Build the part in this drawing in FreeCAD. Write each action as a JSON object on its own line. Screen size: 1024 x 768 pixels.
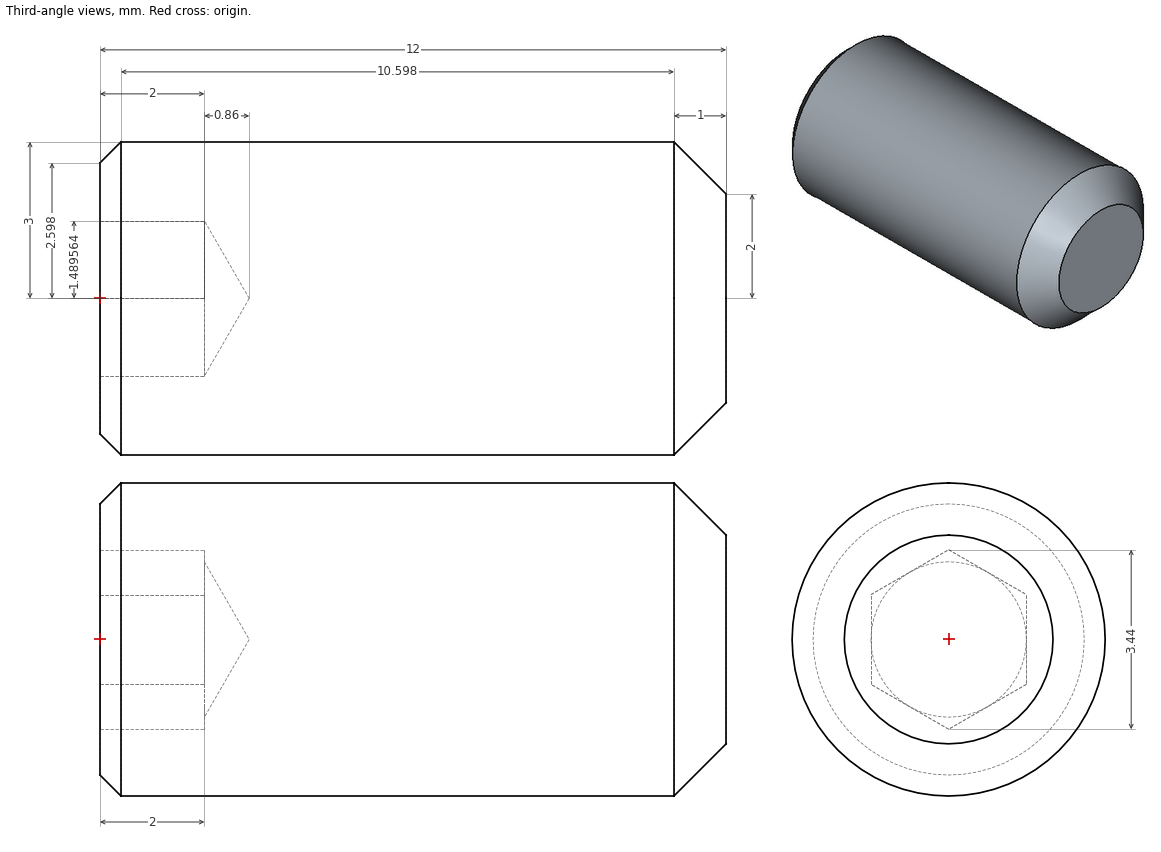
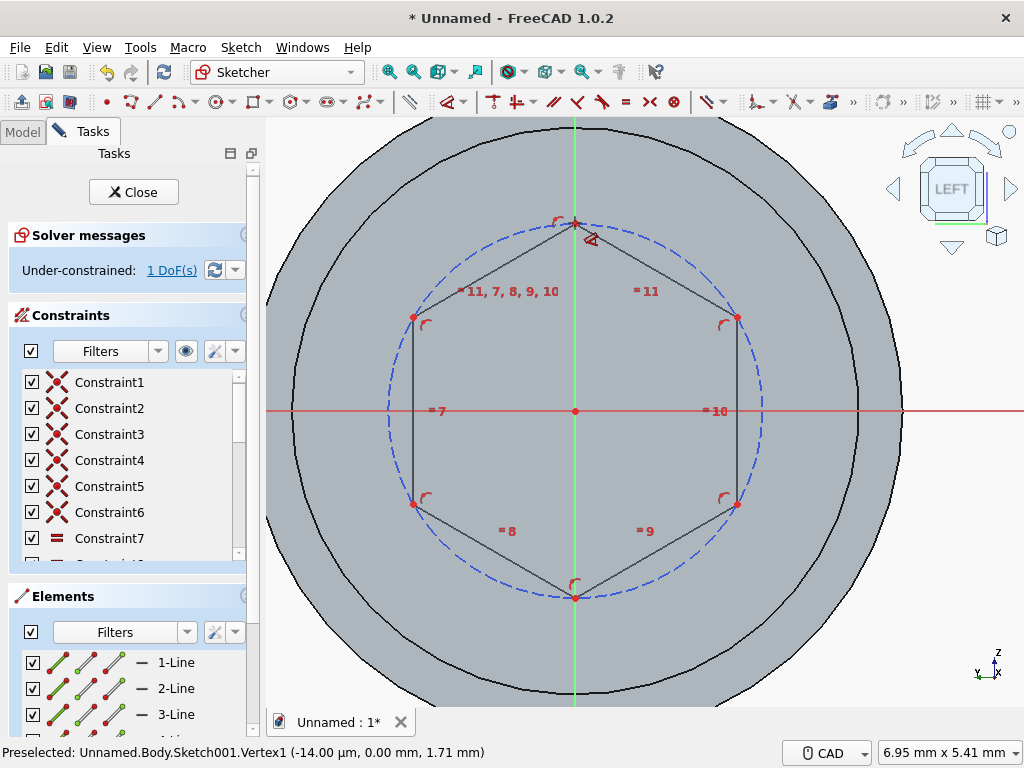
{"action": "left_click", "coordinate": [575, 598]}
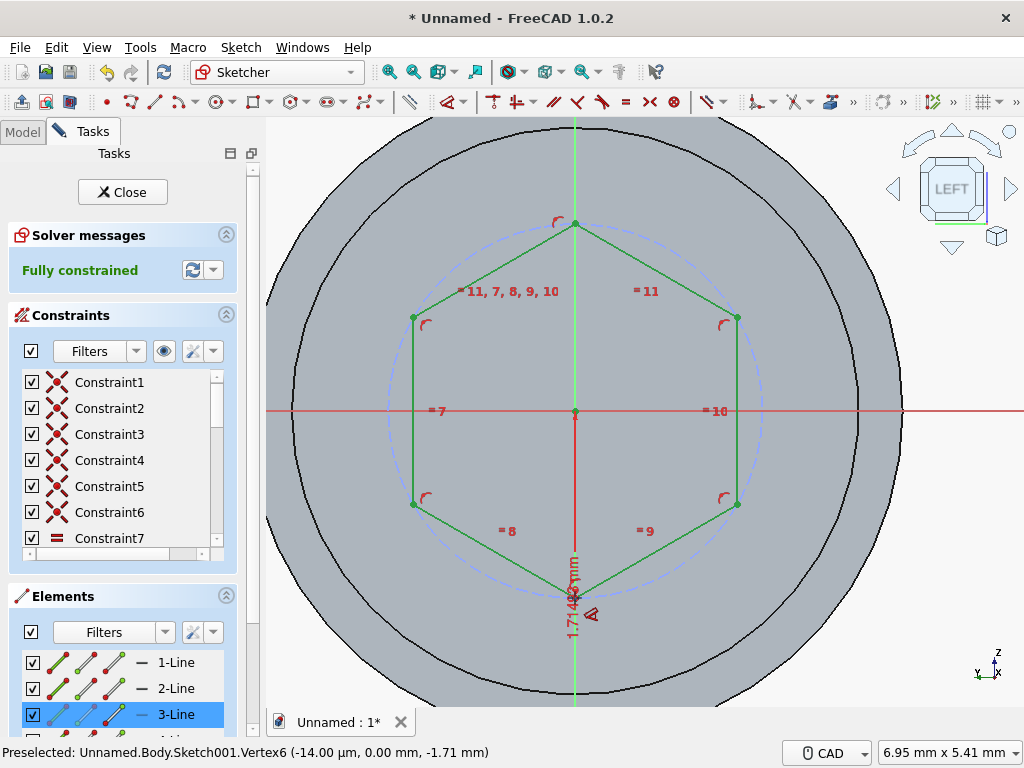
{"action": "left_click", "coordinate": [575, 224]}
{"action": "left_click", "coordinate": [609, 325]}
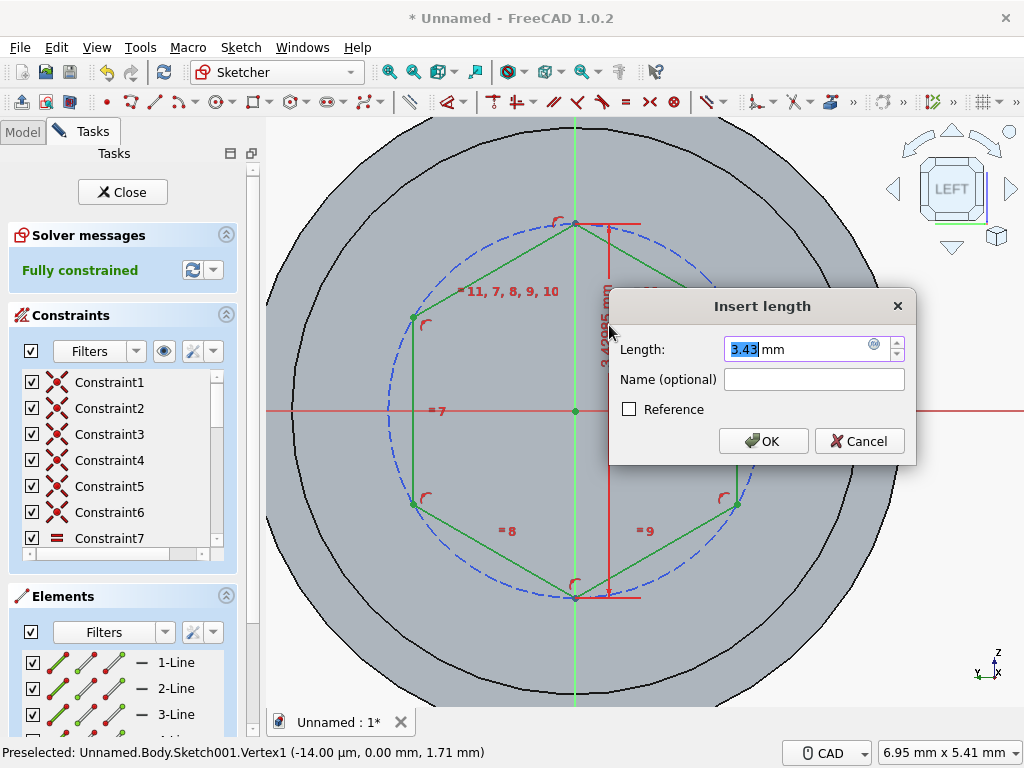
{"action": "type", "text": "3.44"}
{"action": "key", "text": "Return"}
{"action": "key", "text": "Escape"}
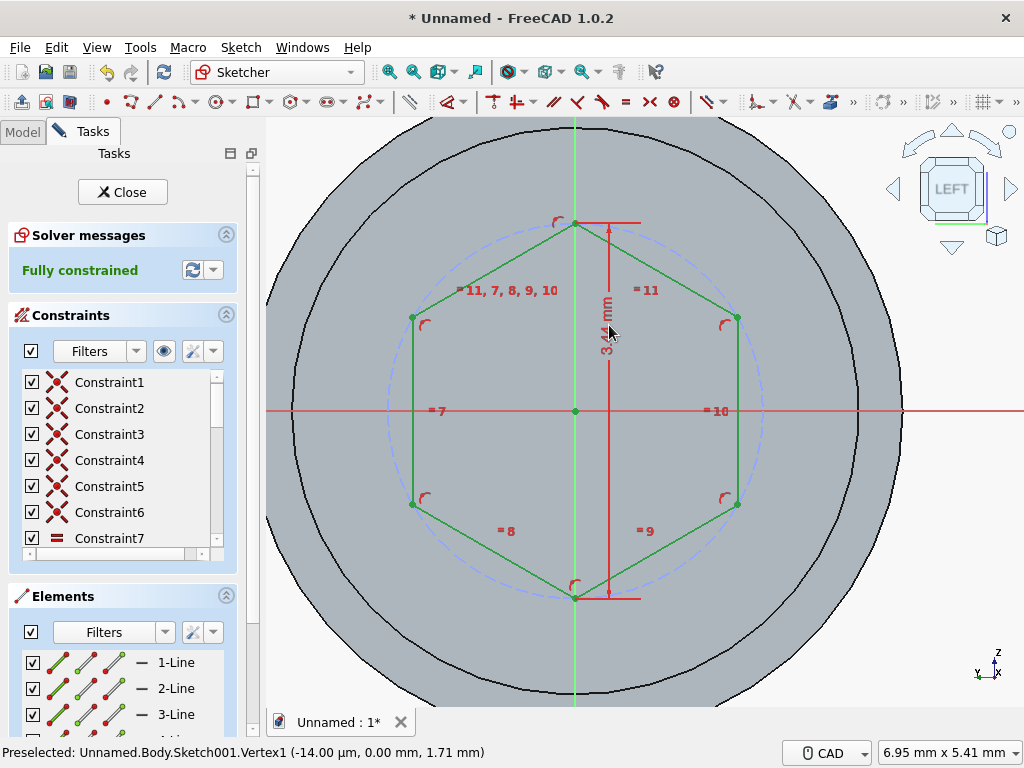
{"action": "left_click", "coordinate": [123, 192]}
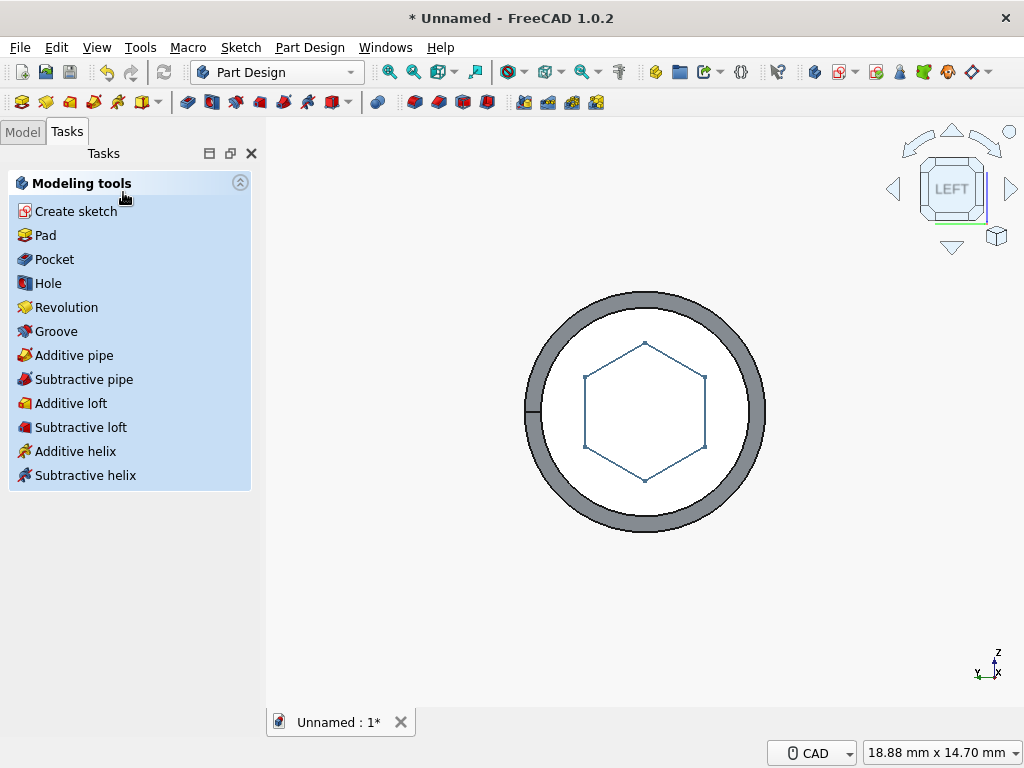
{"action": "left_click", "coordinate": [188, 102]}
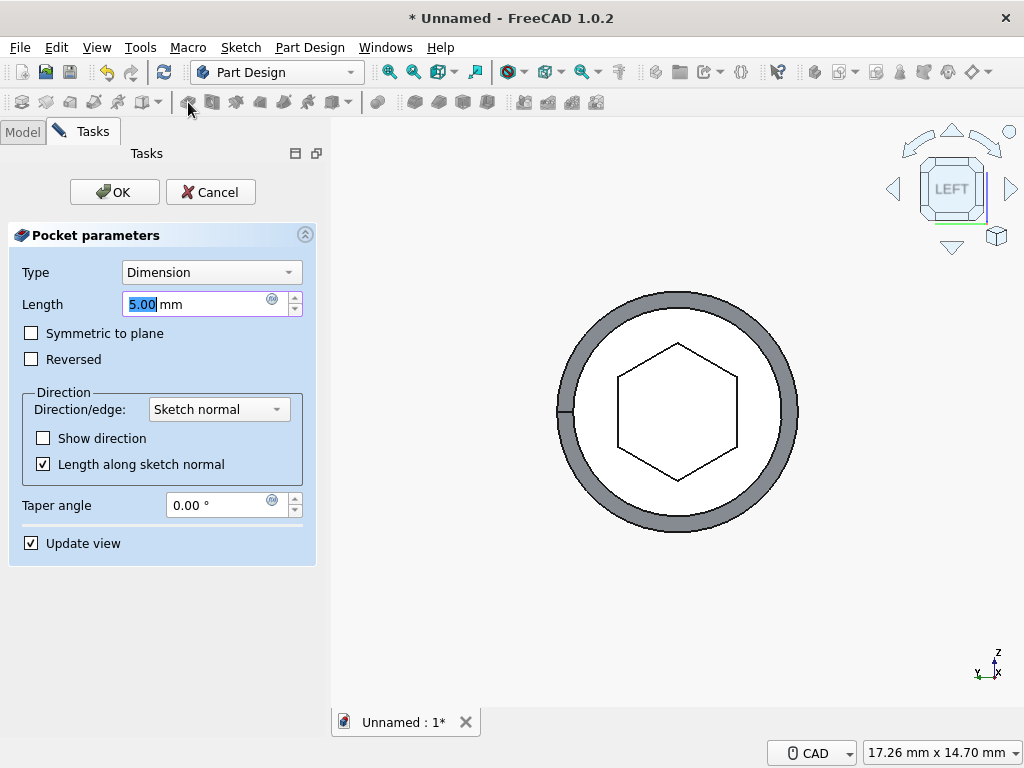
{"action": "type", "text": "2"}
{"action": "key", "text": "Tab"}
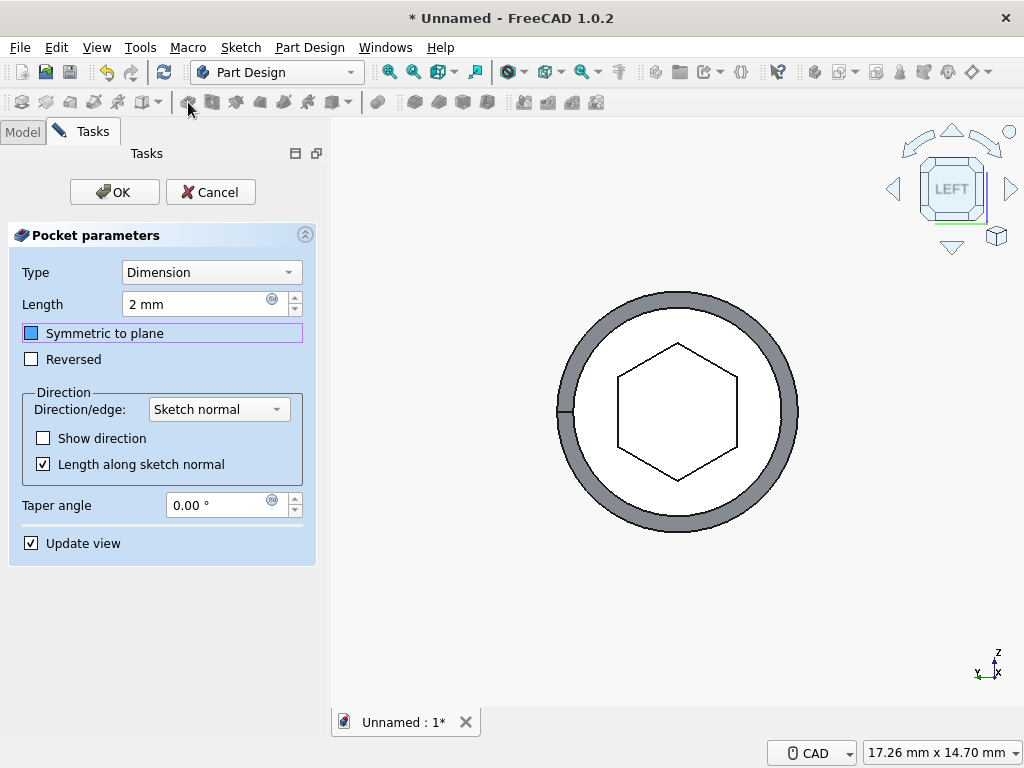
{"action": "left_click", "coordinate": [115, 192]}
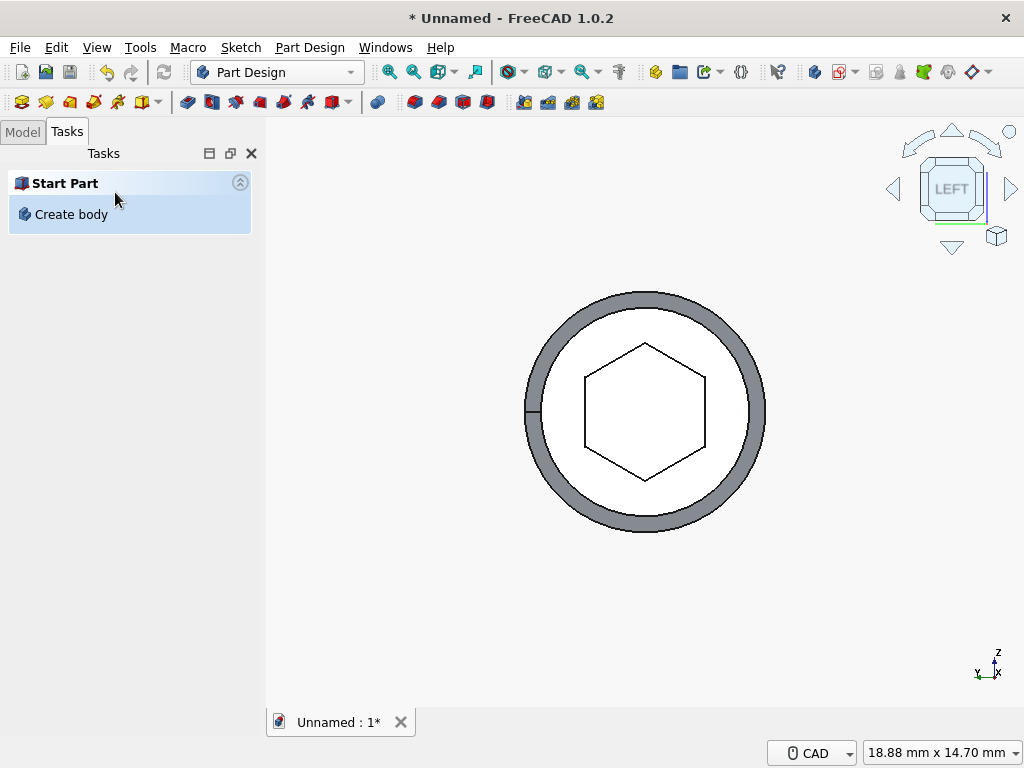
{"action": "left_click", "coordinate": [390, 72]}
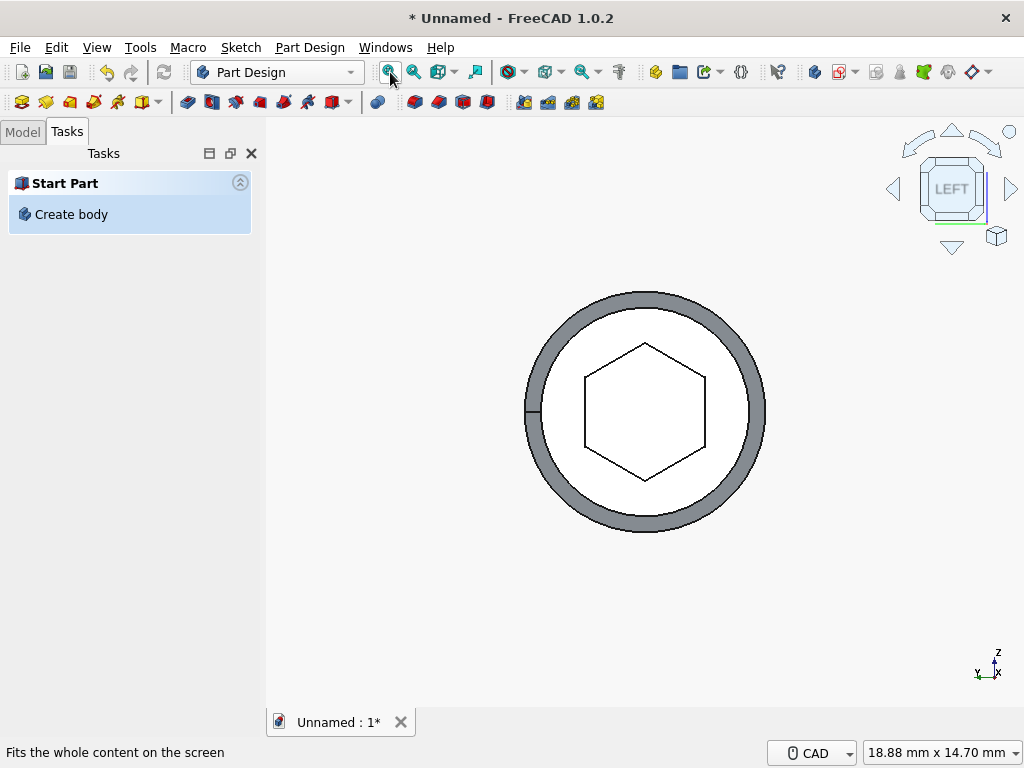
{"action": "left_click", "coordinate": [840, 72]}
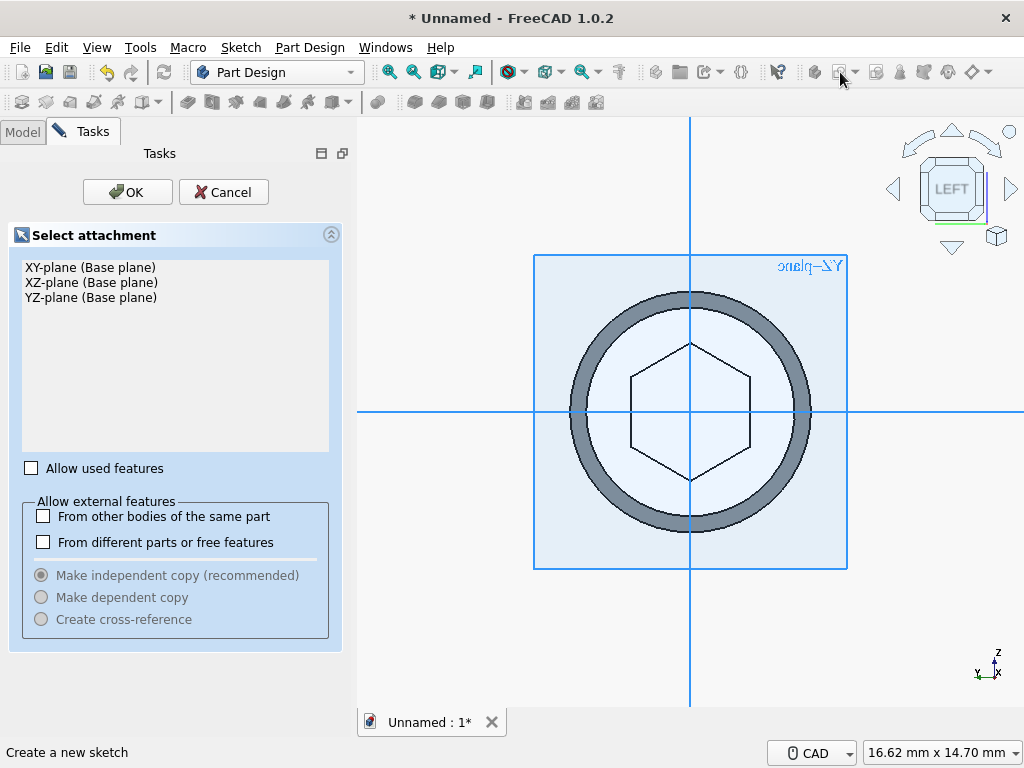
{"action": "left_click", "coordinate": [82, 268]}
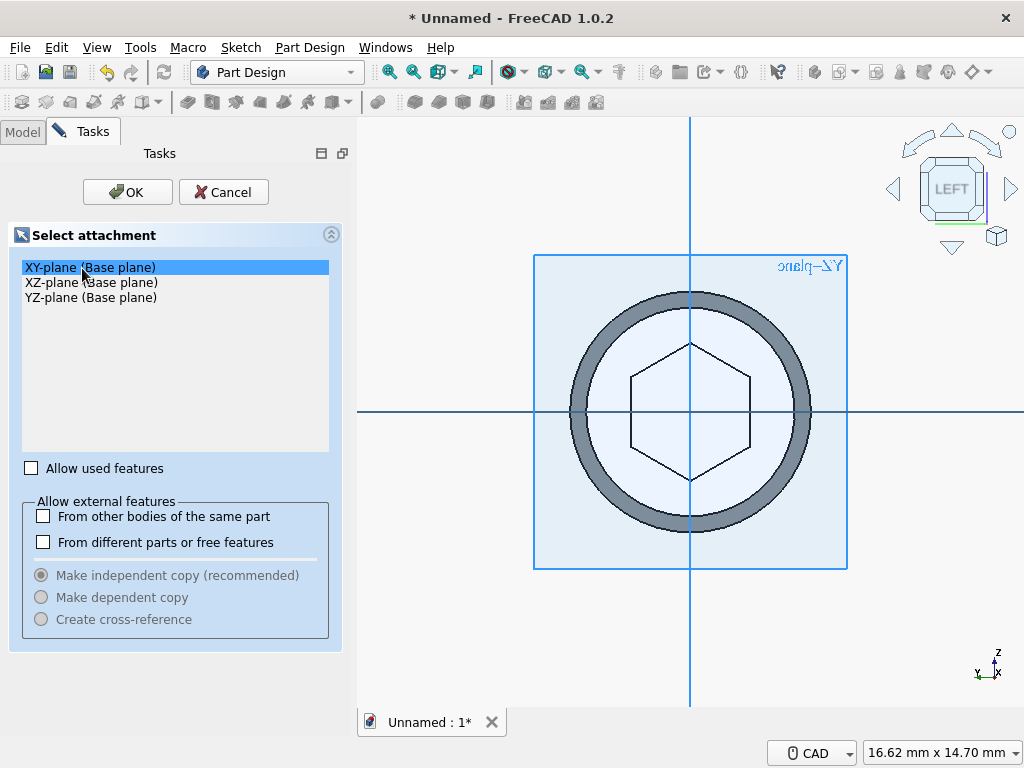
{"action": "left_click", "coordinate": [128, 192]}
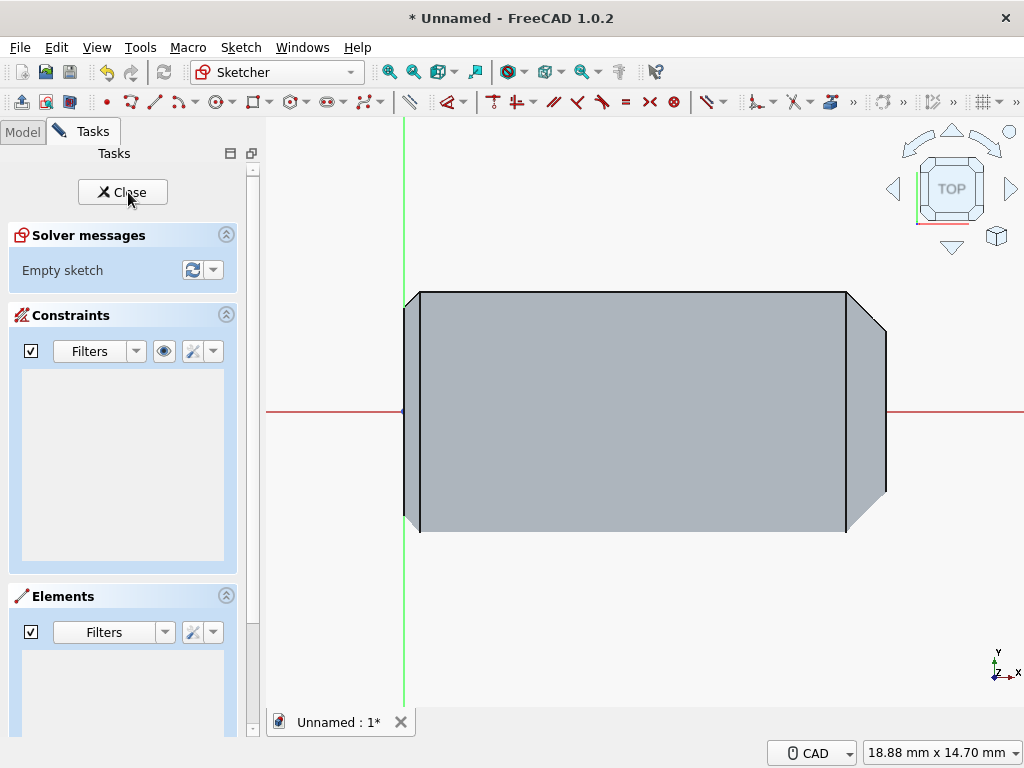
{"action": "key", "text": "q s"}